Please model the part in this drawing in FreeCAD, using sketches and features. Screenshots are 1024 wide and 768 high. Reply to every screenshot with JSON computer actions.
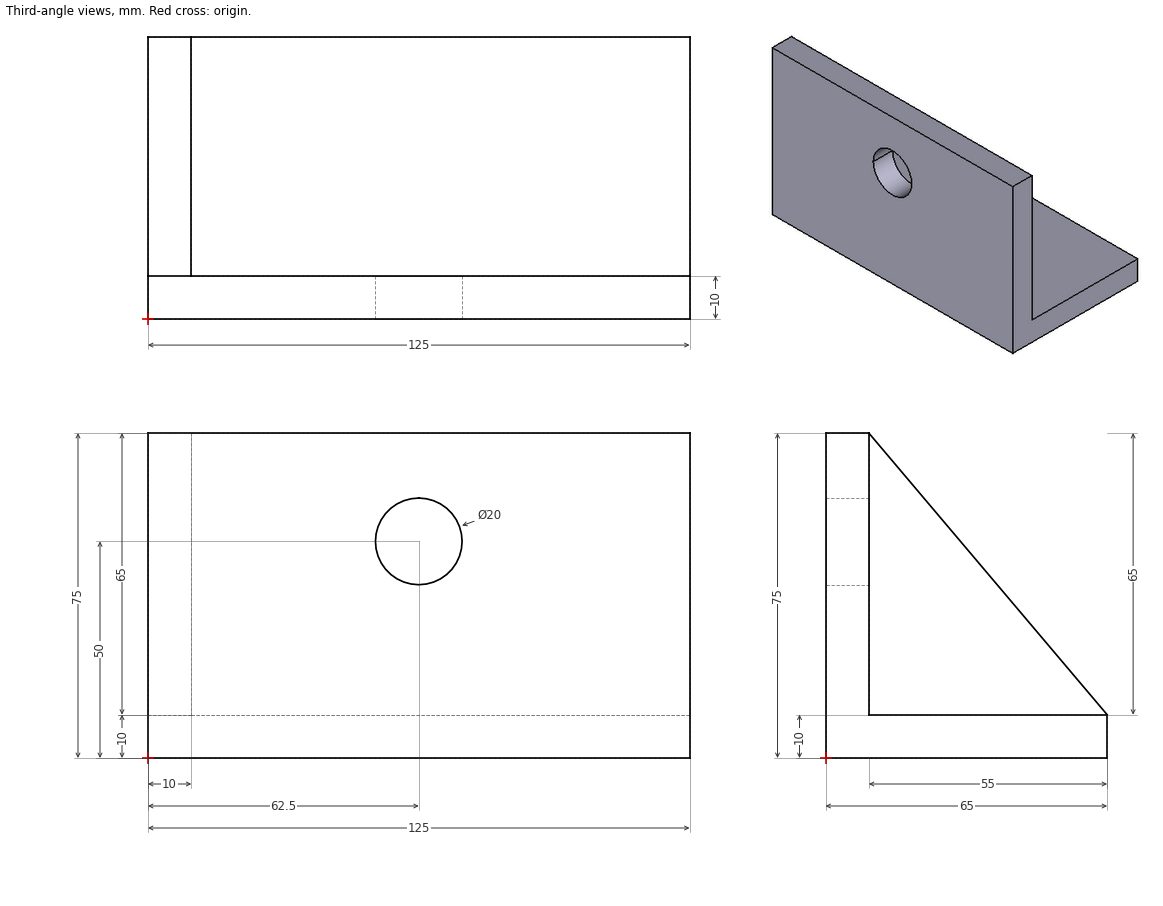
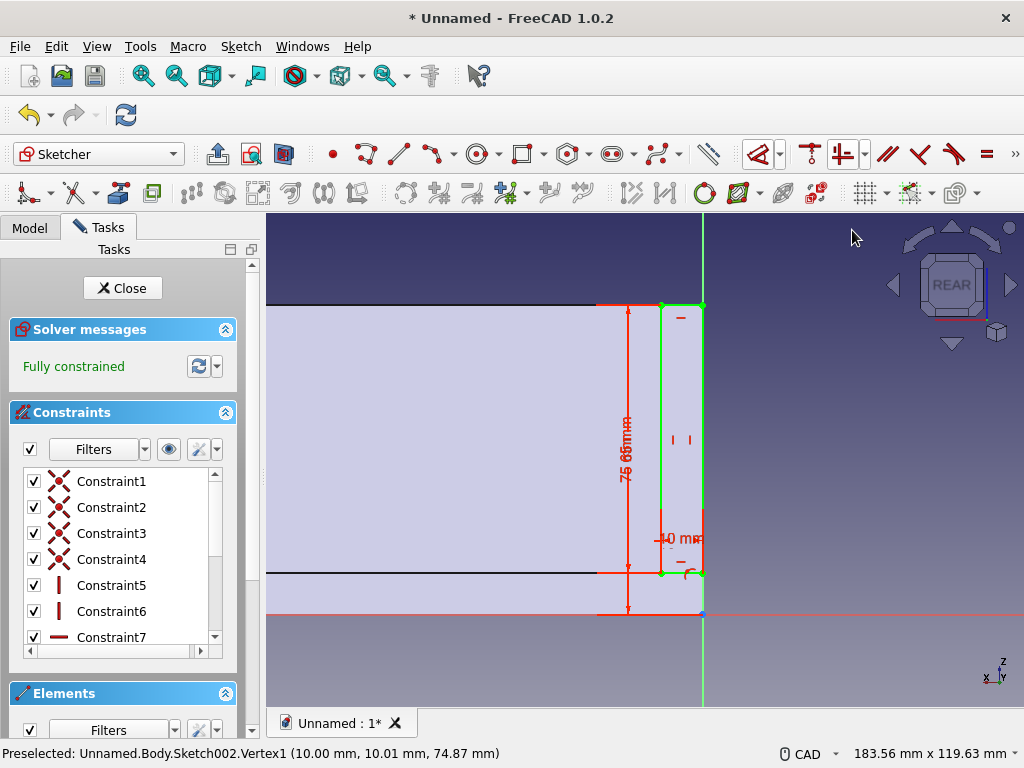
{"action": "left_click", "coordinate": [123, 288]}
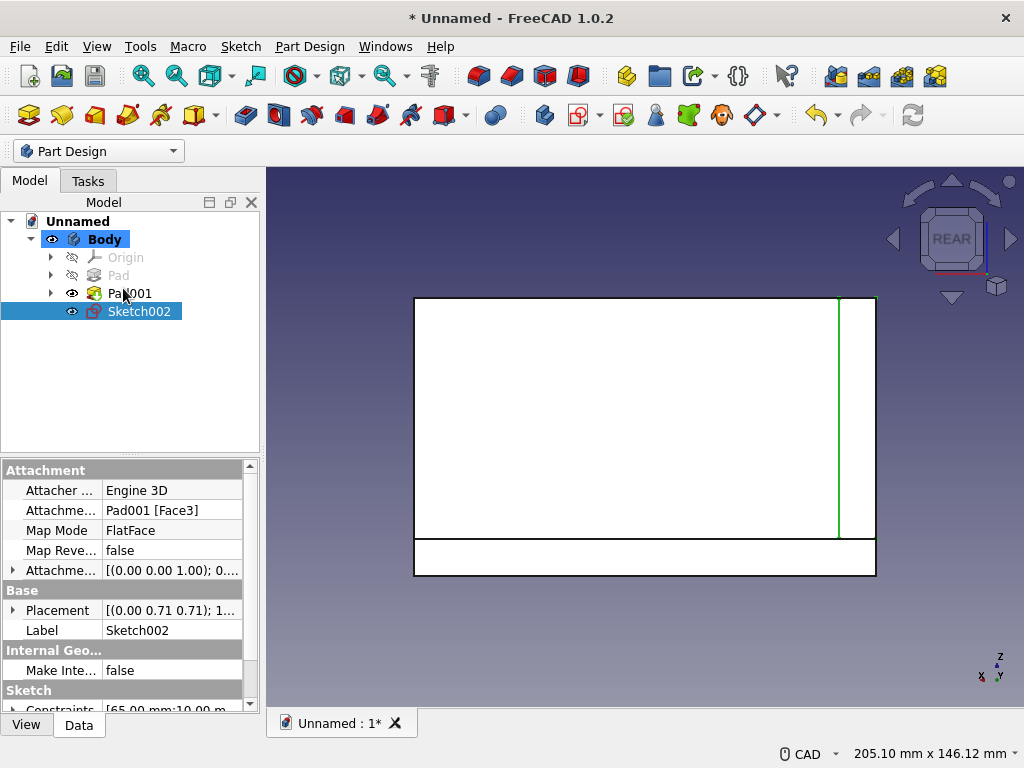
{"action": "left_click", "coordinate": [29, 116]}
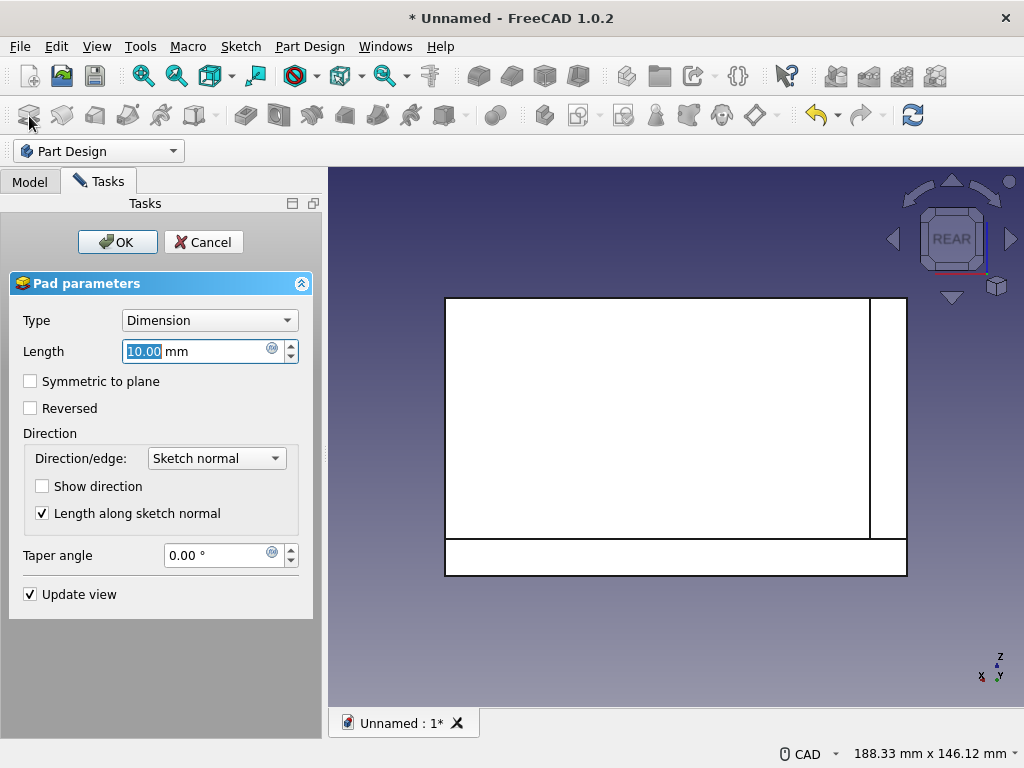
{"action": "type", "text": "55"}
{"action": "key", "text": "Tab"}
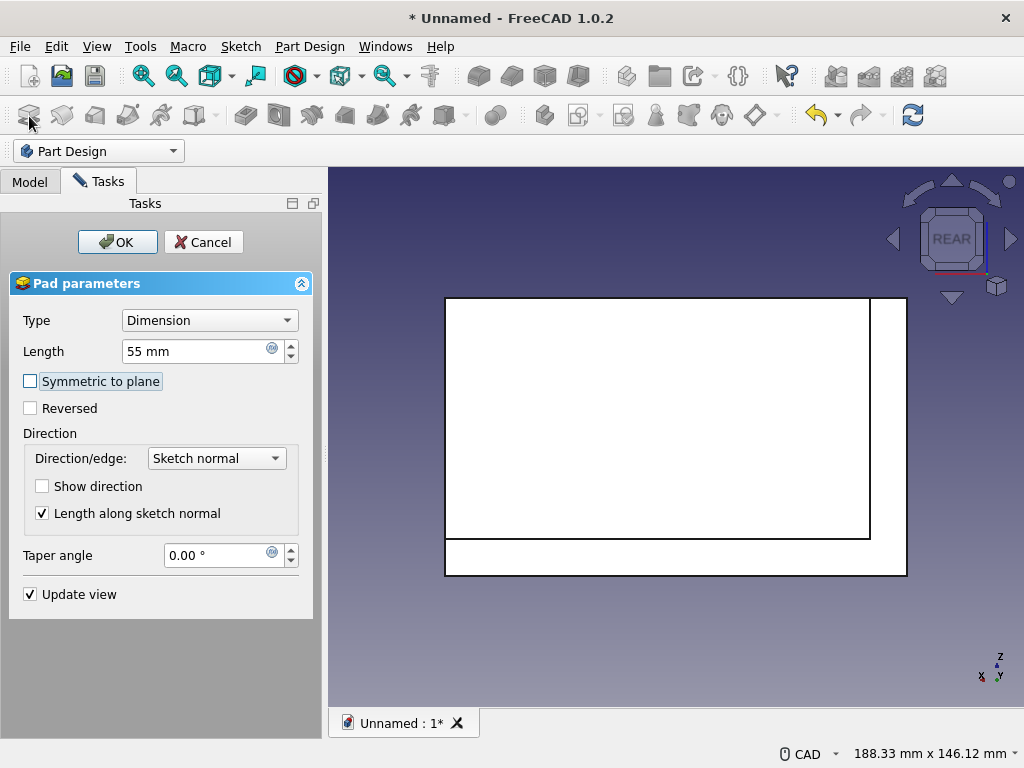
{"action": "left_click", "coordinate": [118, 242]}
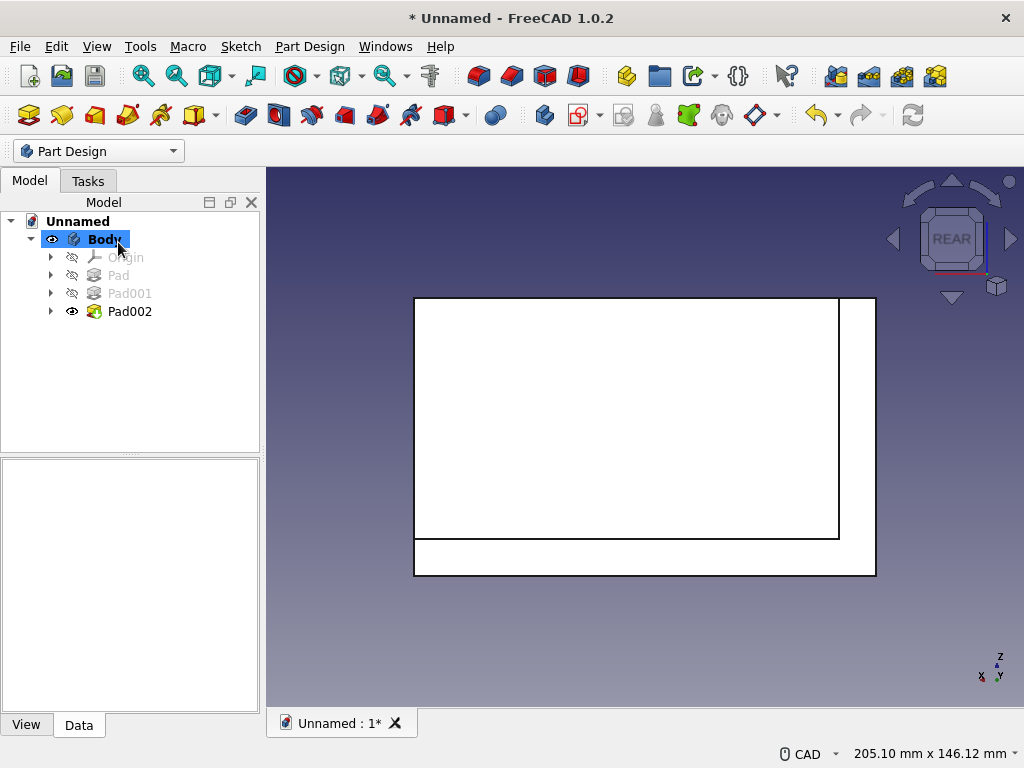
{"action": "key", "text": "0"}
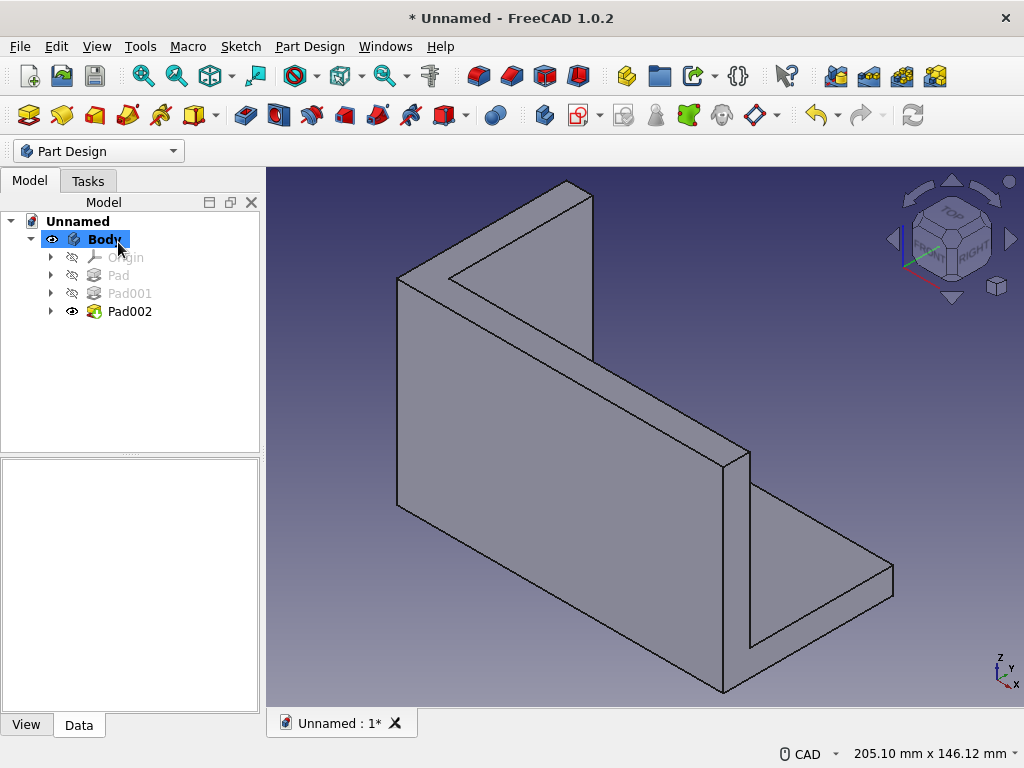
{"action": "left_click", "coordinate": [521, 306]}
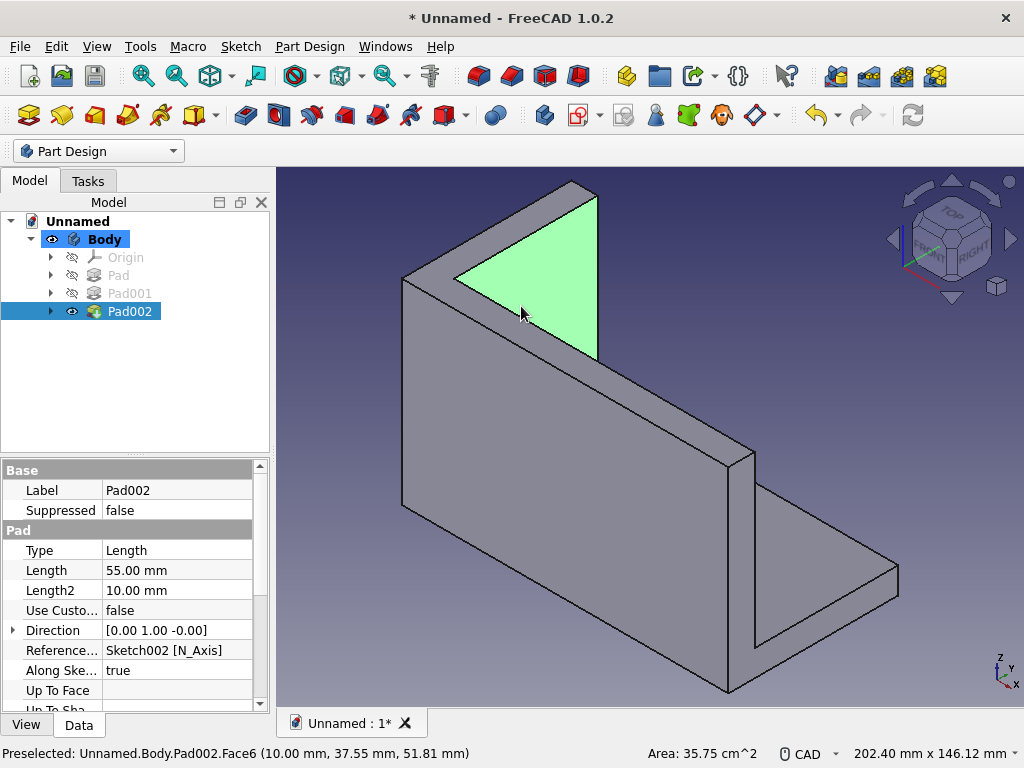
{"action": "left_click", "coordinate": [578, 116]}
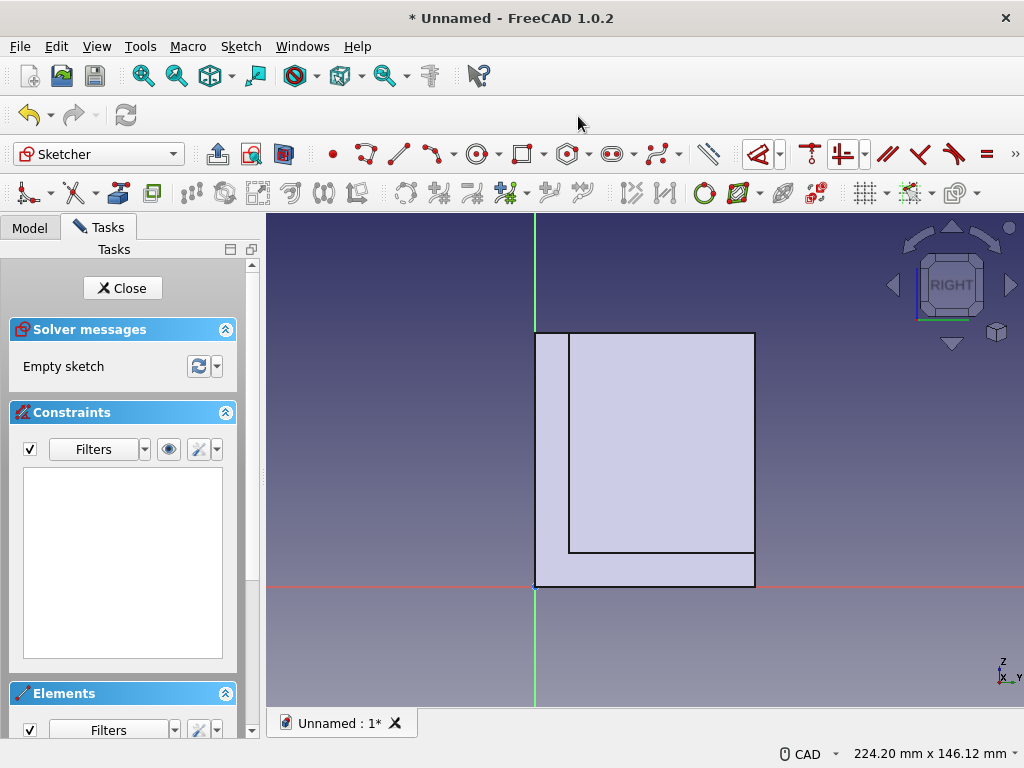
{"action": "left_click", "coordinate": [366, 154]}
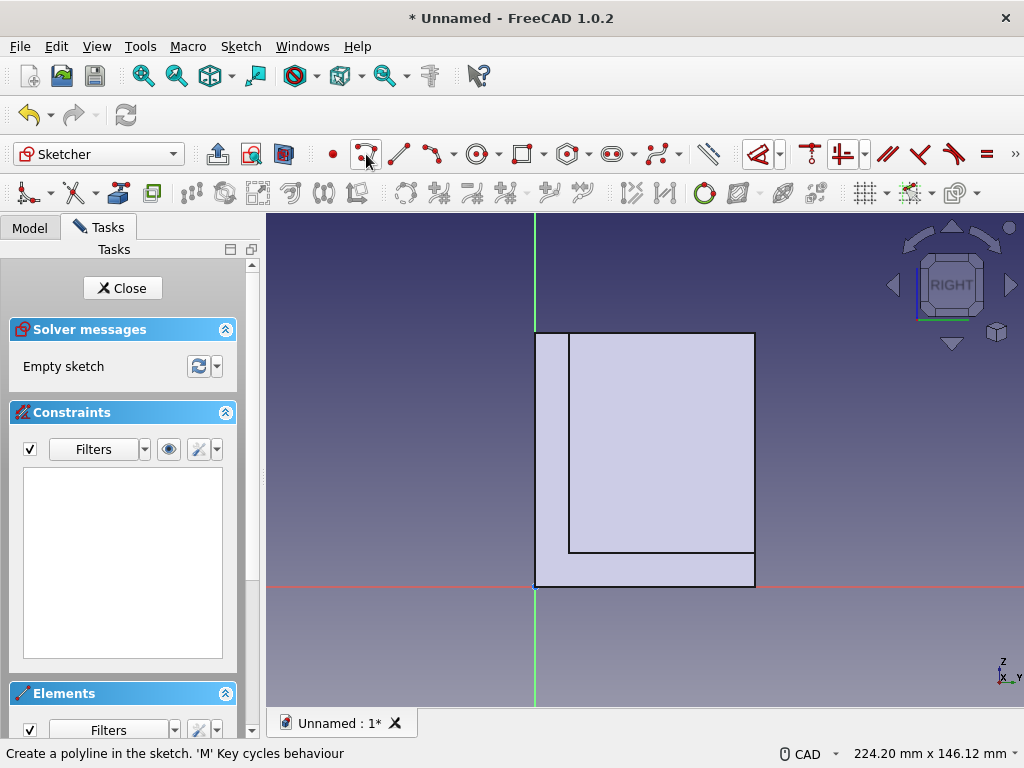
{"action": "left_click", "coordinate": [755, 553]}
{"action": "left_click", "coordinate": [755, 333]}
{"action": "left_click", "coordinate": [569, 333]}
{"action": "left_click", "coordinate": [755, 554]}
{"action": "key", "text": "Escape"}
{"action": "key", "text": "Escape"}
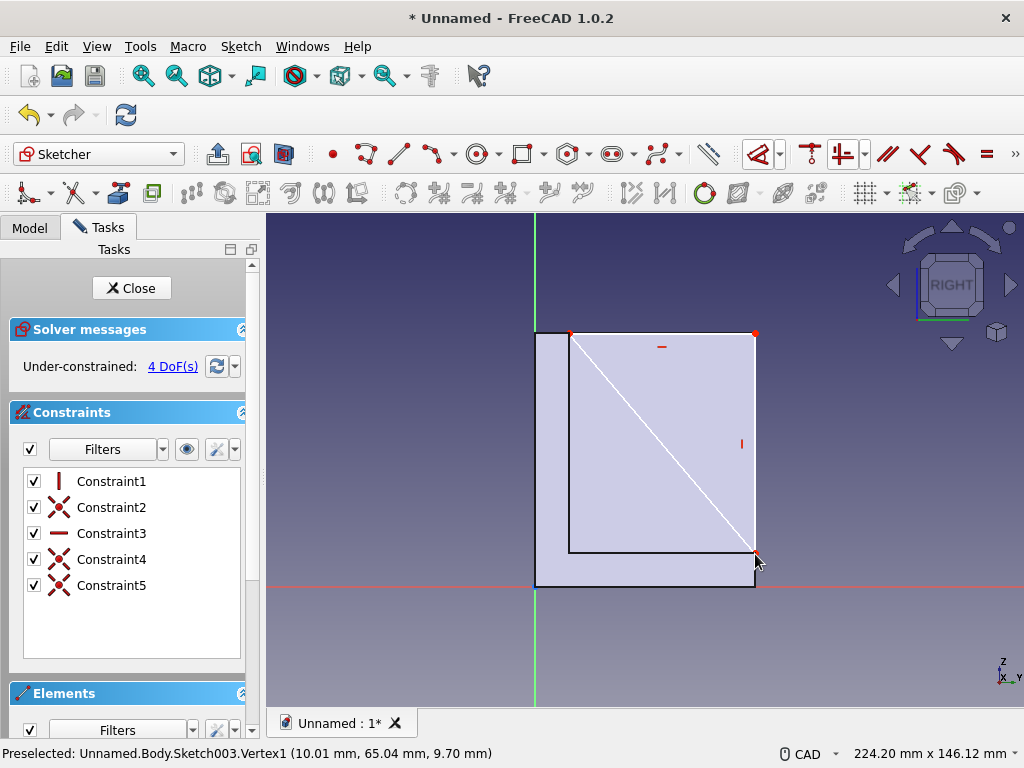
{"action": "left_click", "coordinate": [755, 488]}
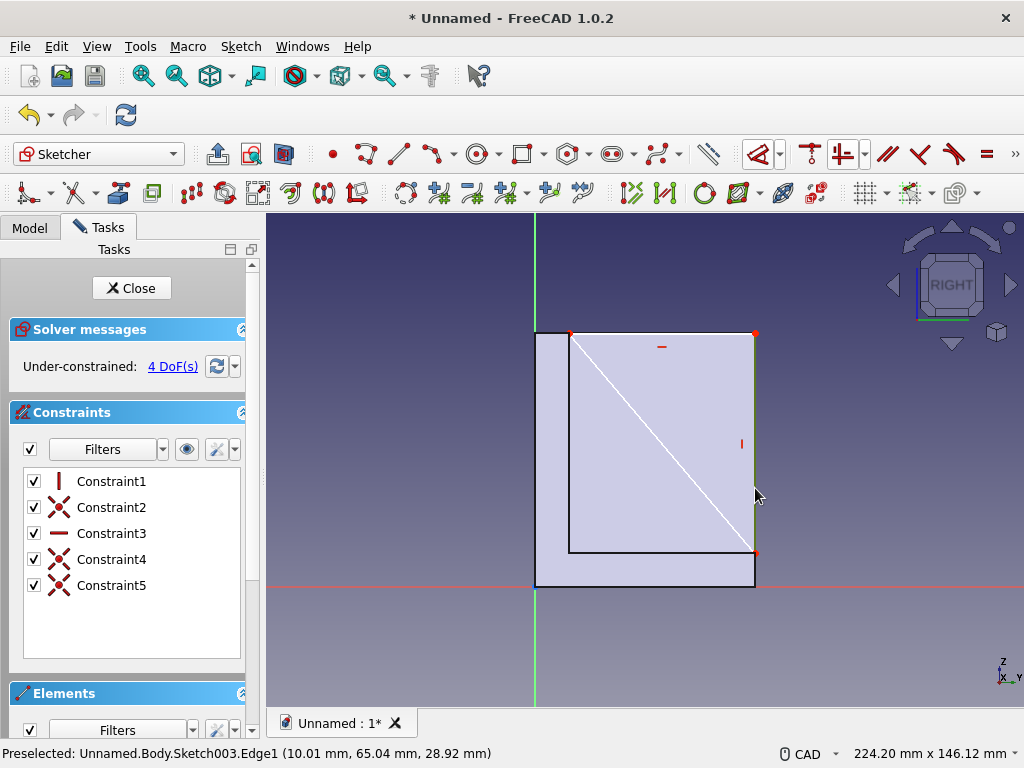
{"action": "key", "text": "i"}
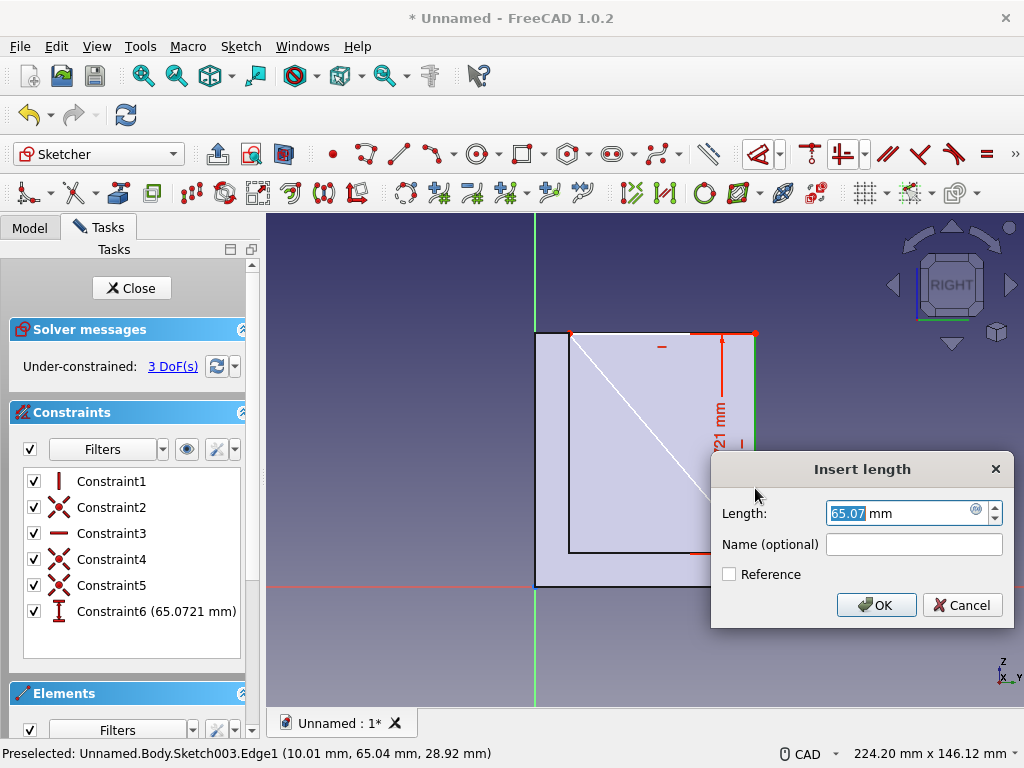
{"action": "type", "text": "65"}
{"action": "key", "text": "Return"}